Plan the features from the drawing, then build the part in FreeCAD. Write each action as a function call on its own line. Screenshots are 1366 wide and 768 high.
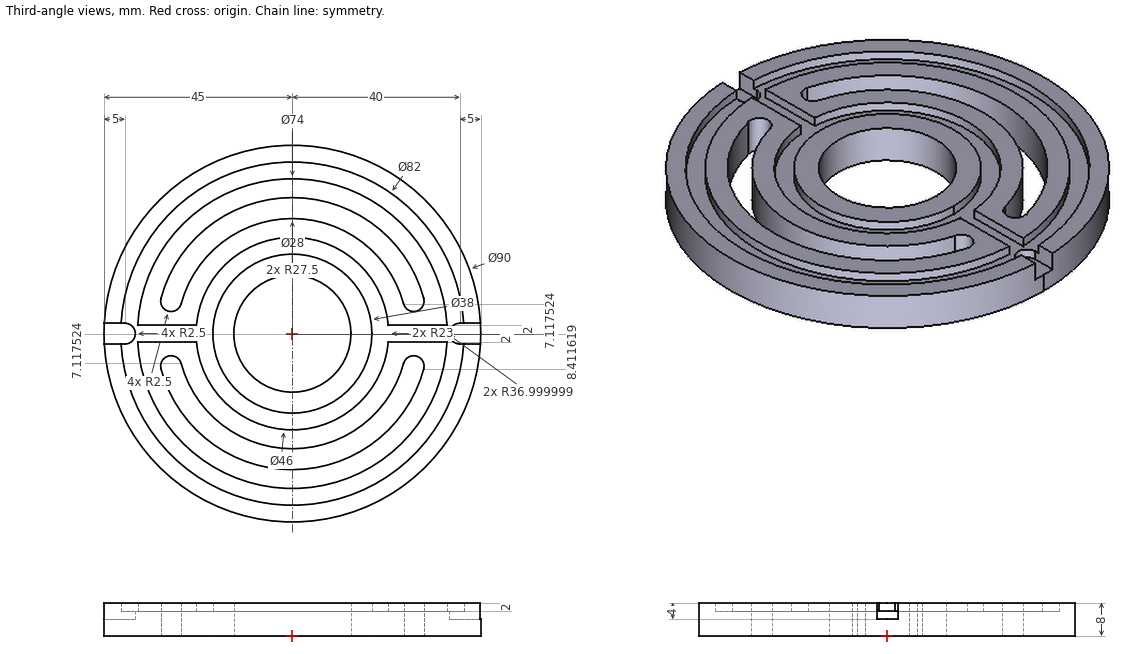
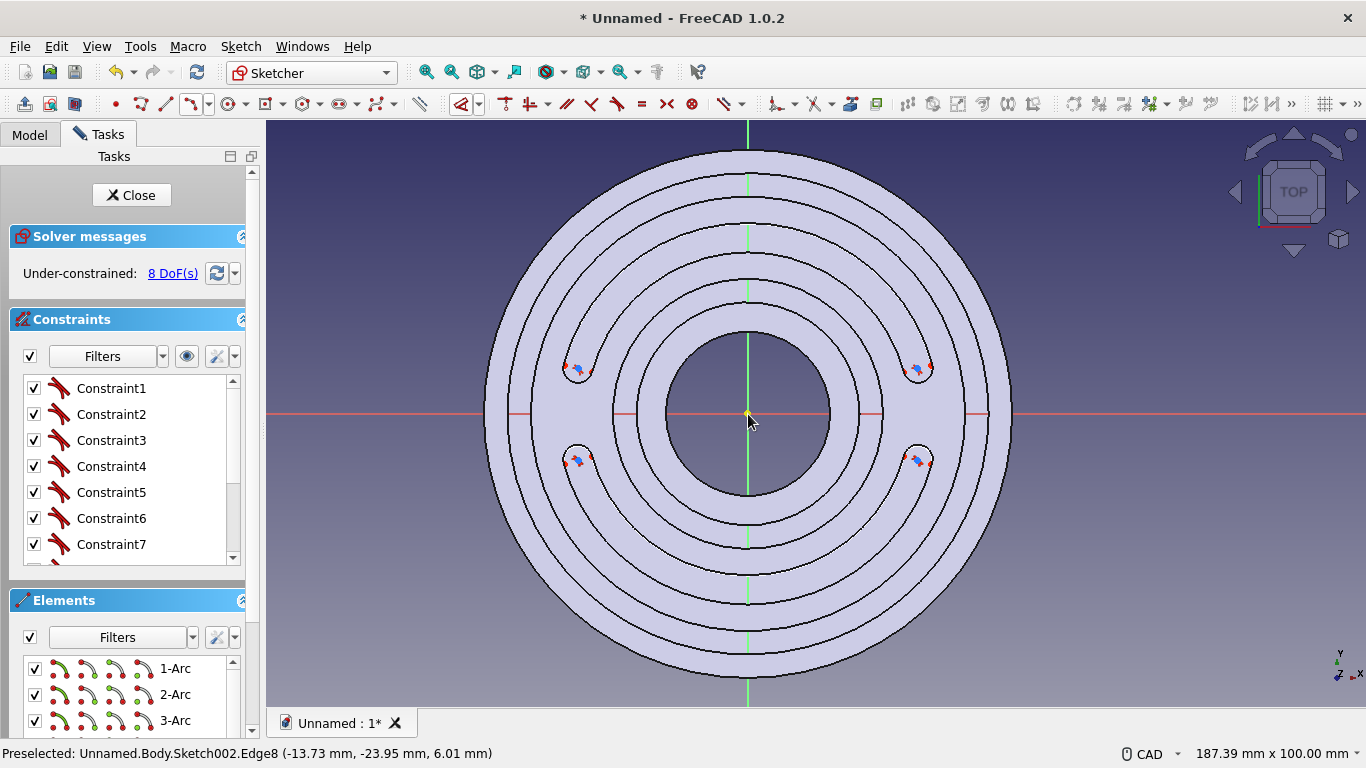
click(913, 382)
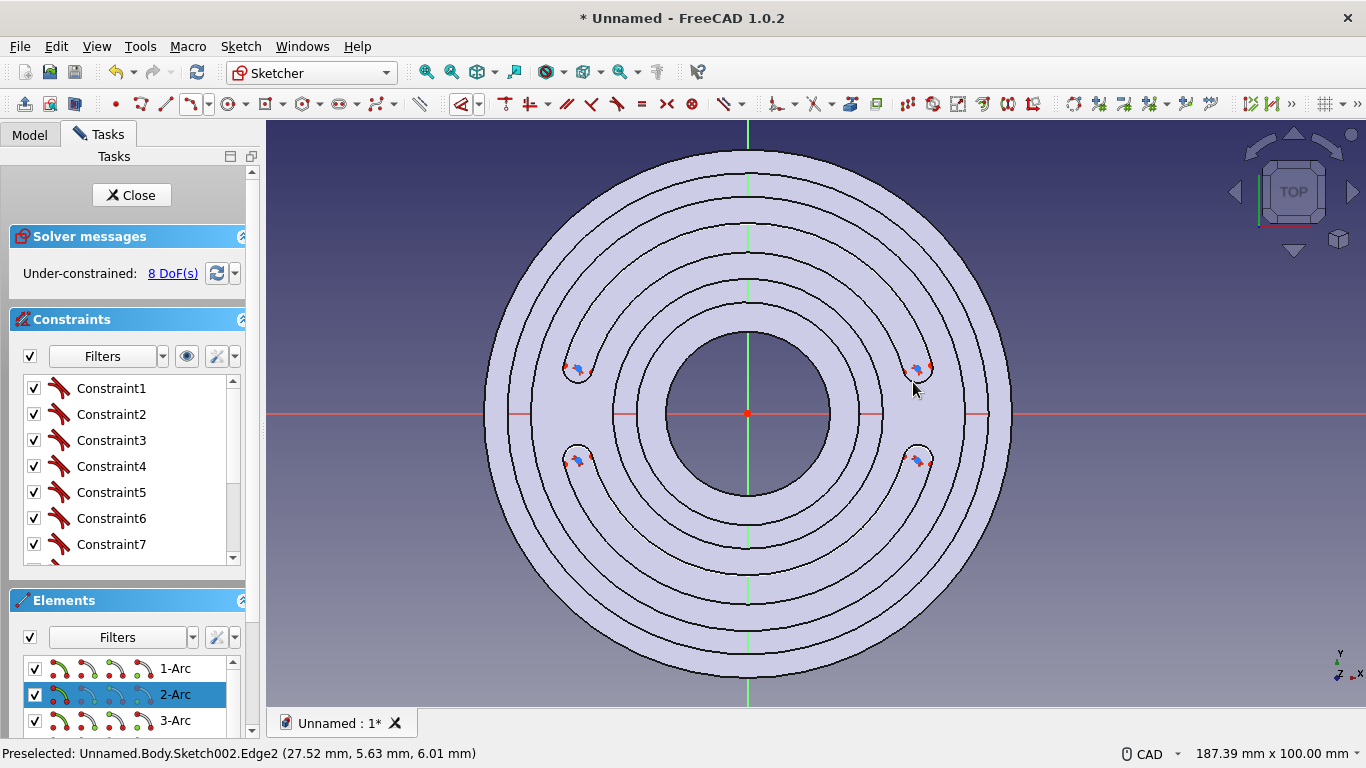
click(583, 447)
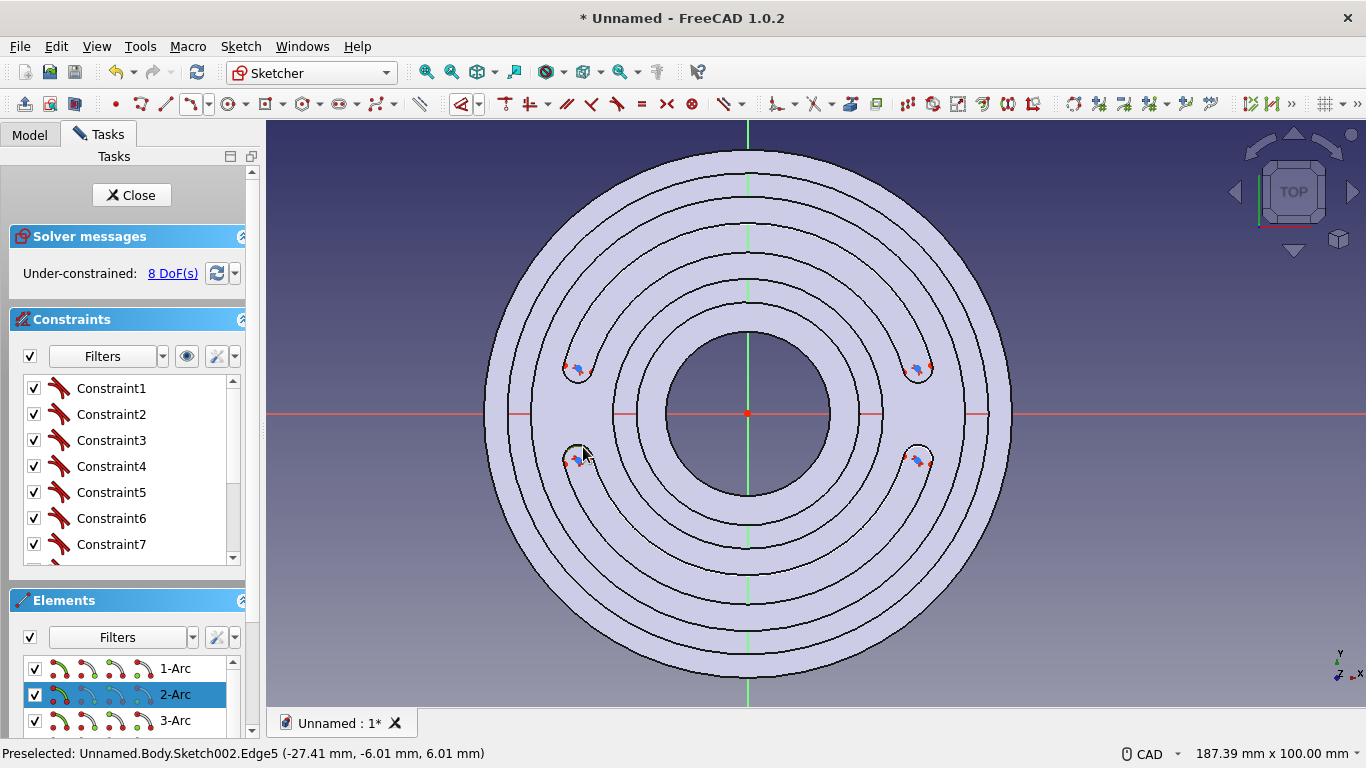
key(e)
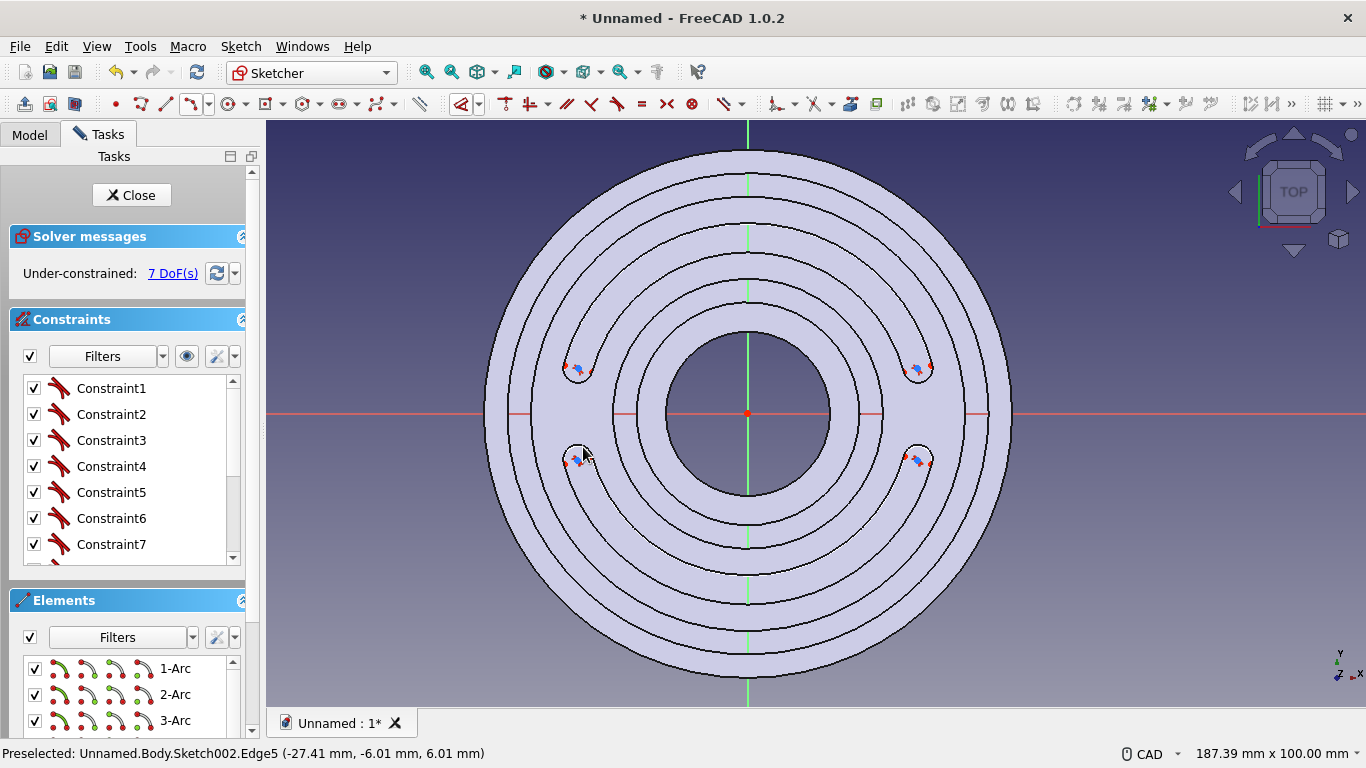
click(843, 249)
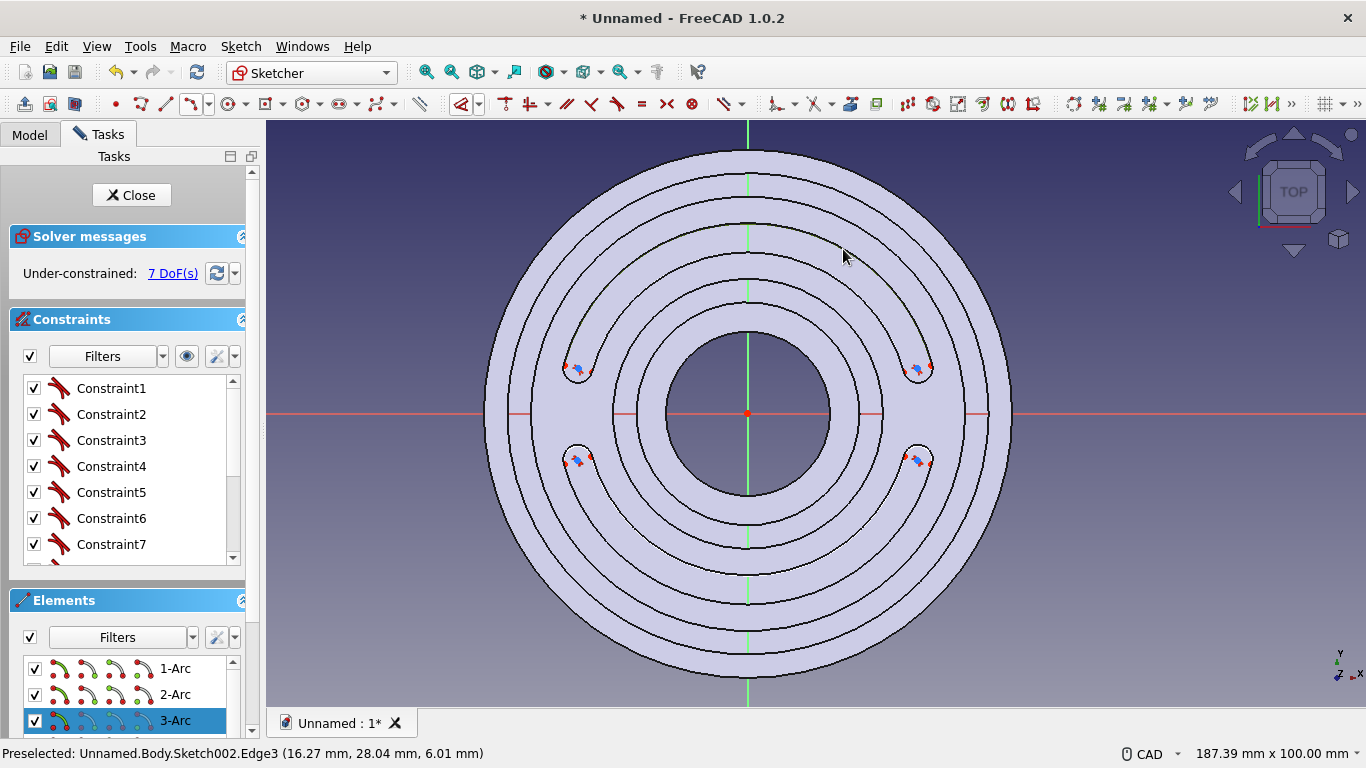
click(653, 579)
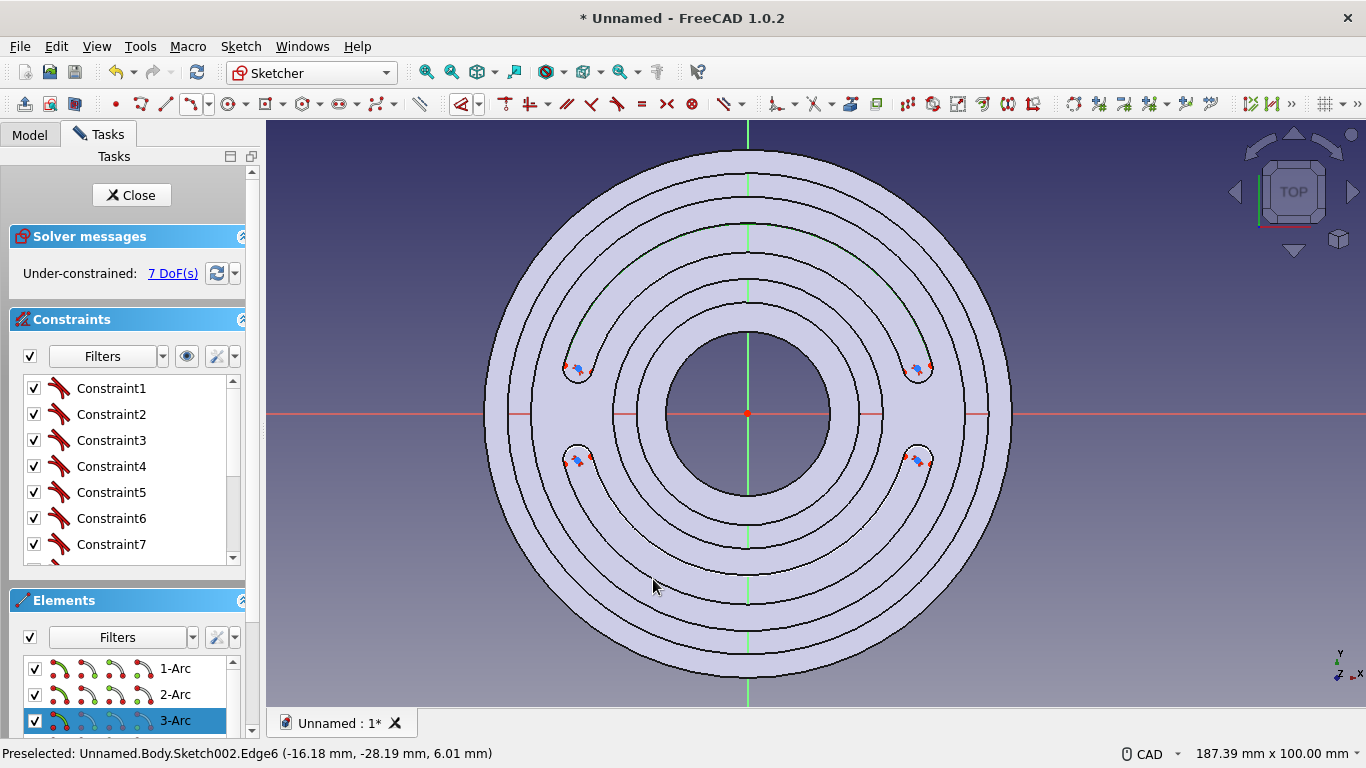
click(642, 104)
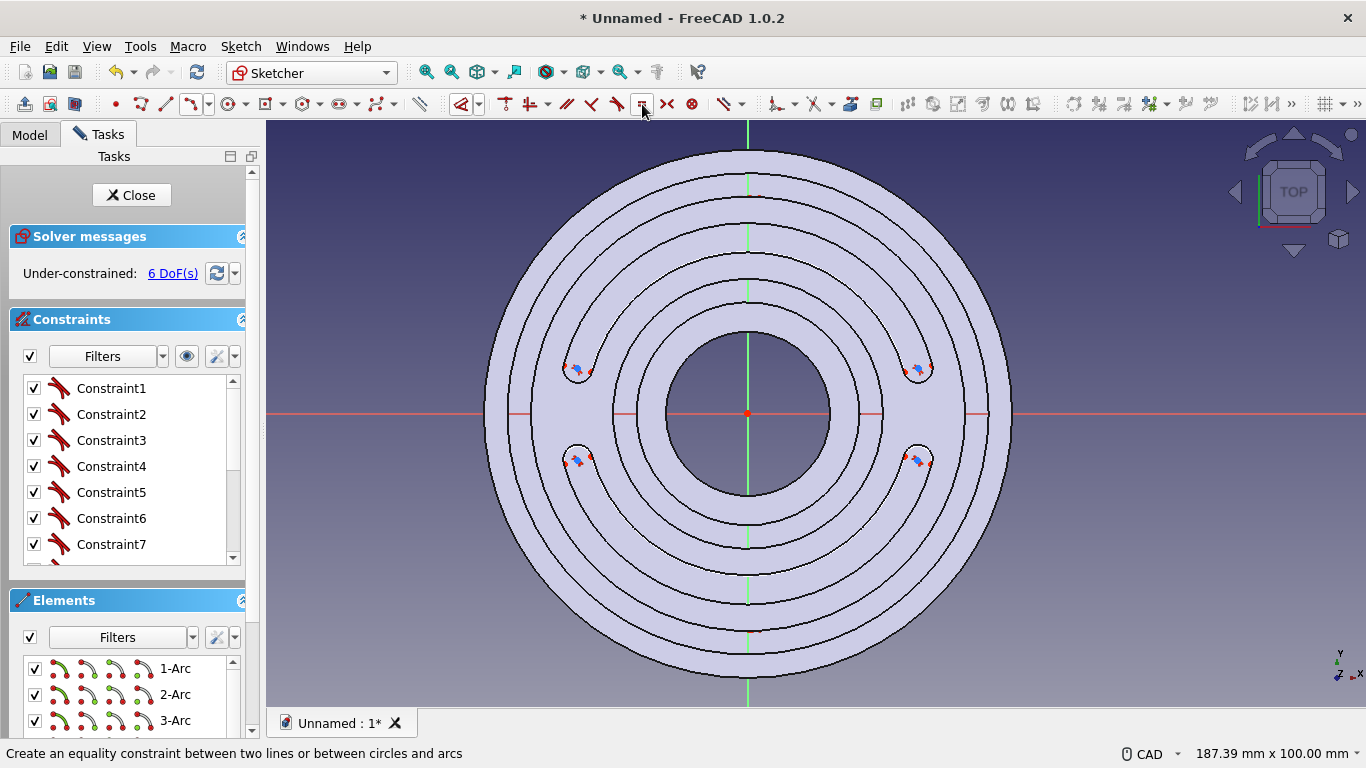
key(d)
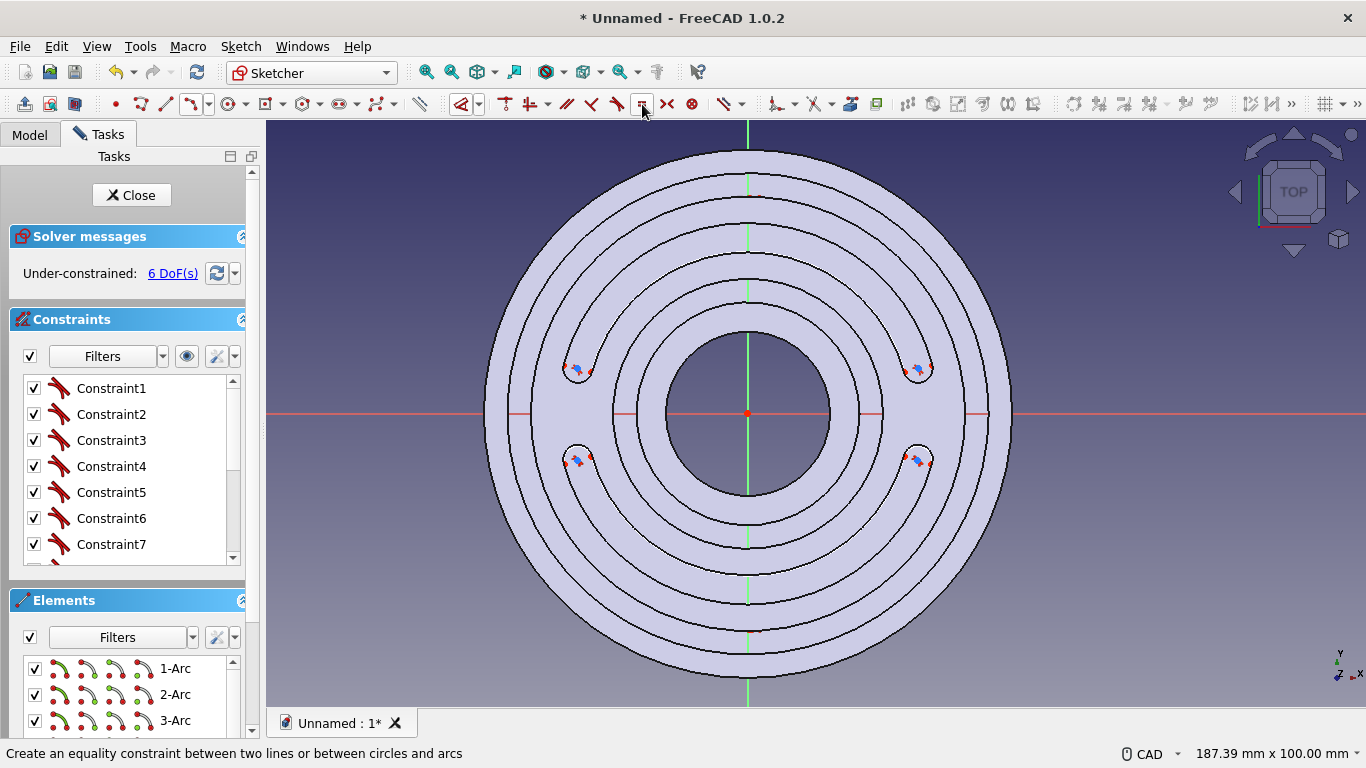
click(829, 274)
click(857, 226)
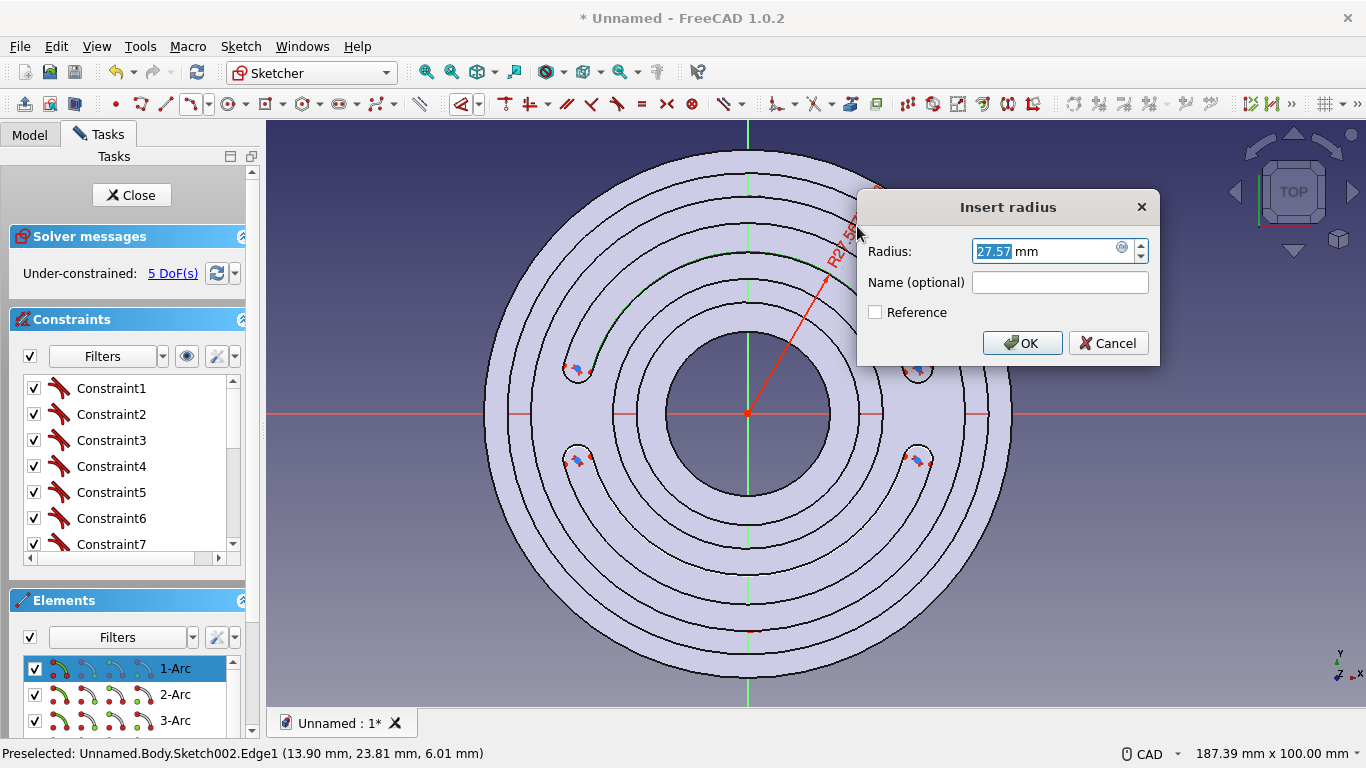
text(27.5)
key(Return)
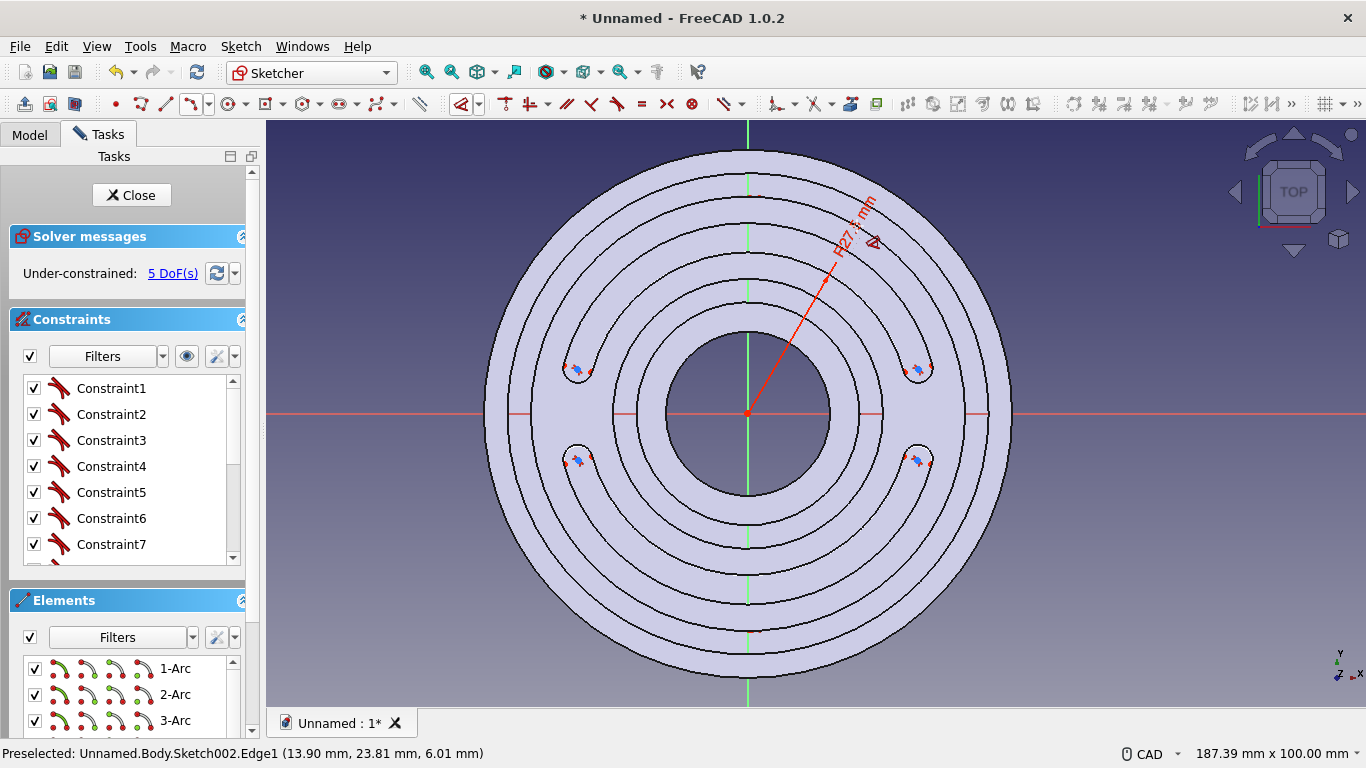
scroll(913, 383, up, 5)